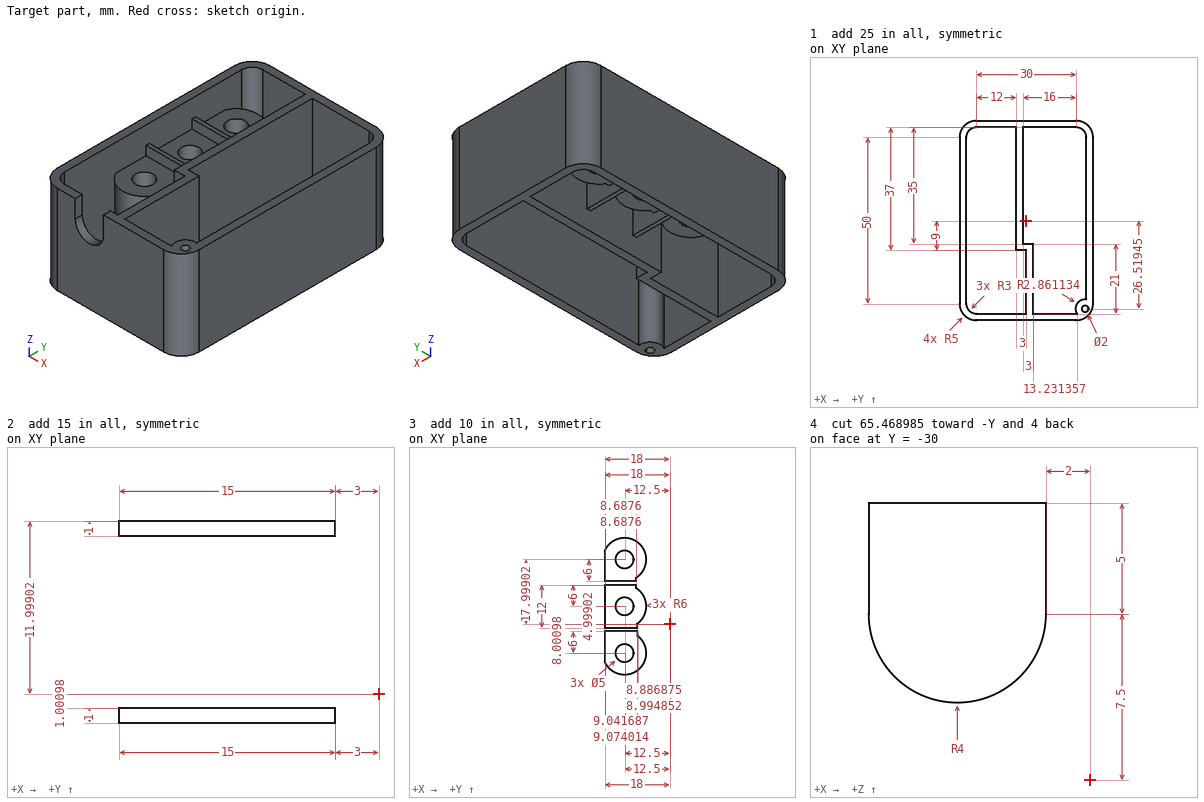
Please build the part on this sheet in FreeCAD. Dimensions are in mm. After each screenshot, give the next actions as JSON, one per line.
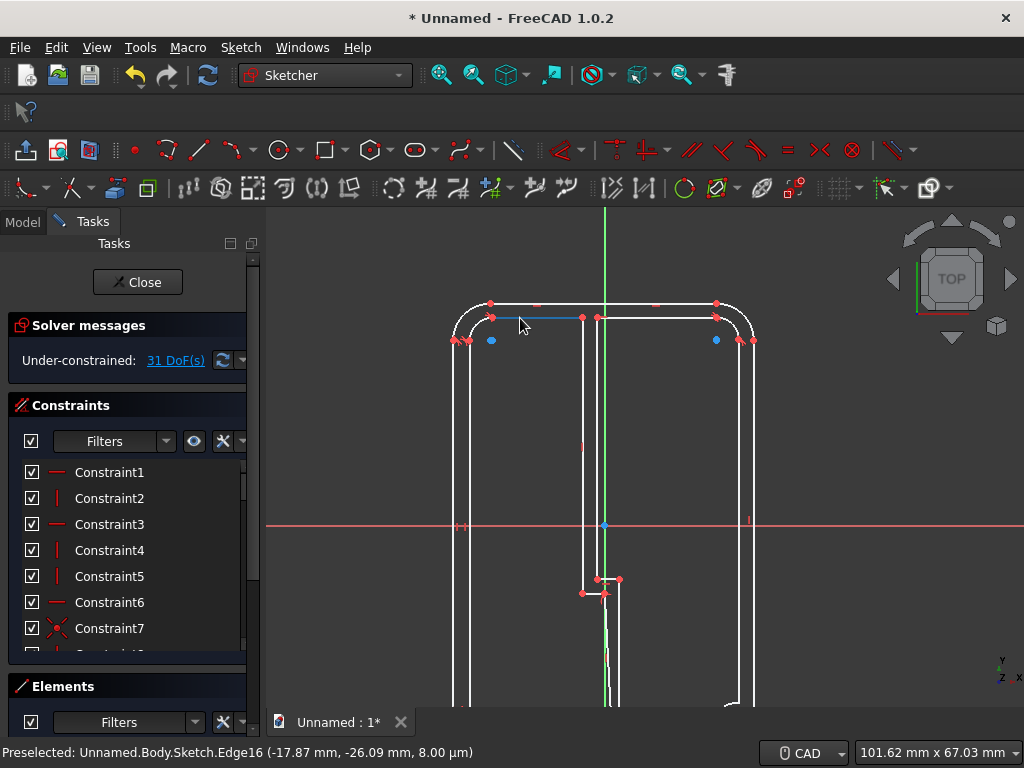
{"action": "left_click", "coordinate": [519, 318]}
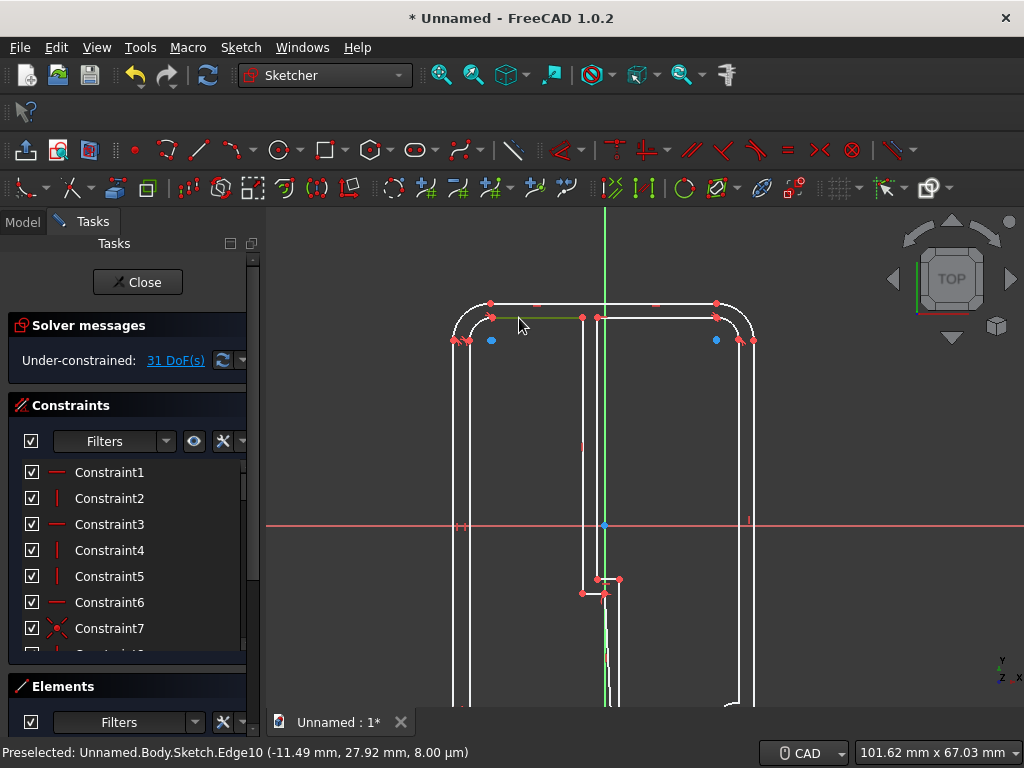
{"action": "scroll", "coordinate": [482, 320], "scroll_direction": "up", "scroll_amount": 2}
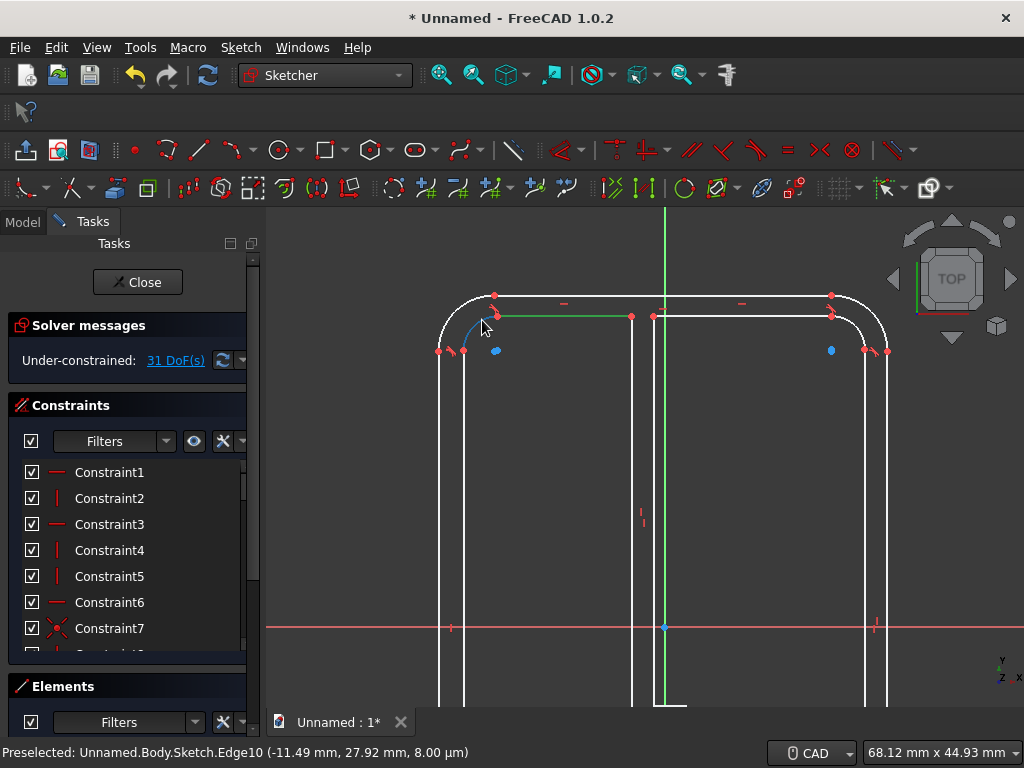
{"action": "left_click", "coordinate": [482, 320]}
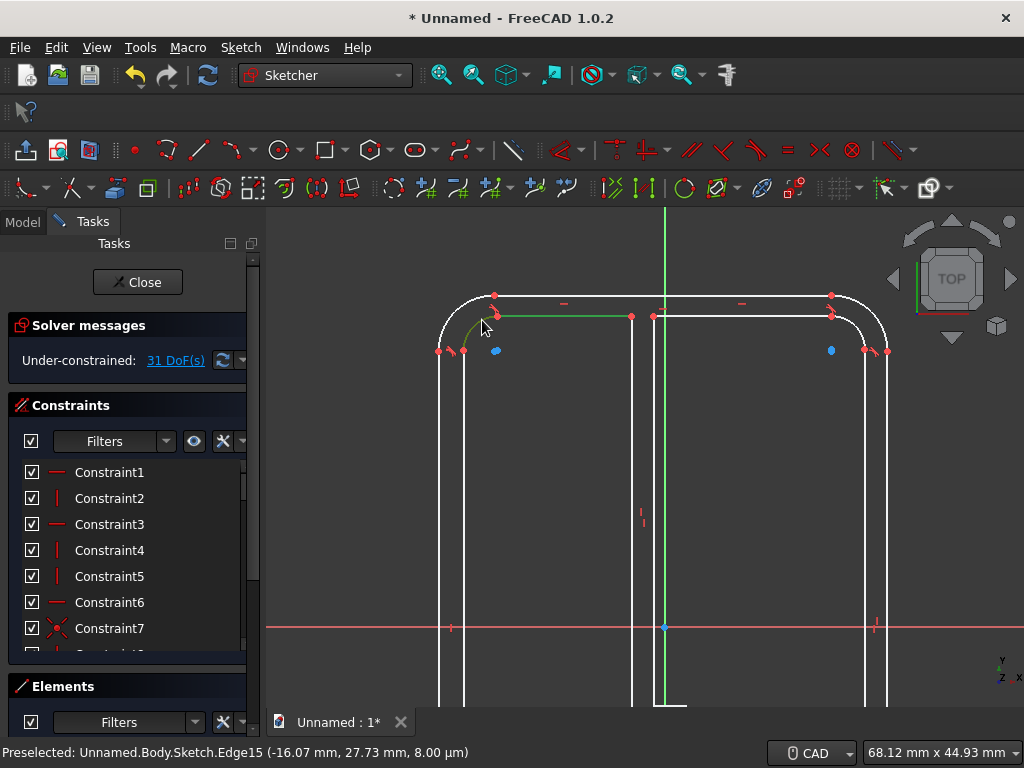
{"action": "left_click", "coordinate": [756, 150]}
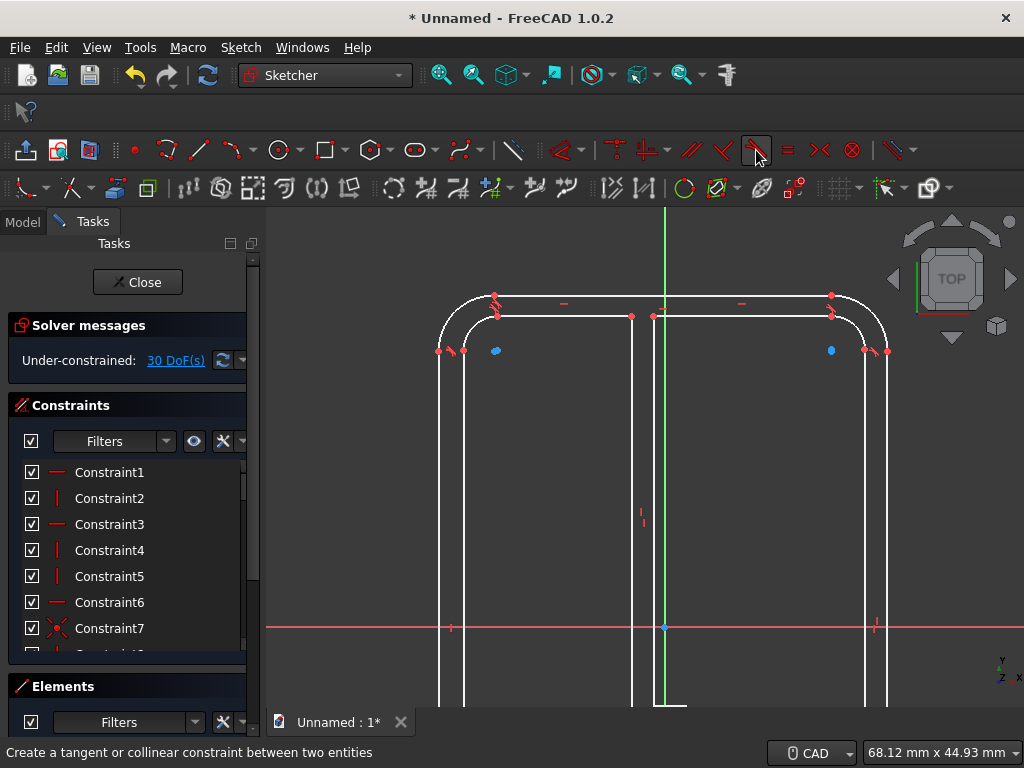
{"action": "scroll", "coordinate": [504, 318], "scroll_direction": "down", "scroll_amount": 4}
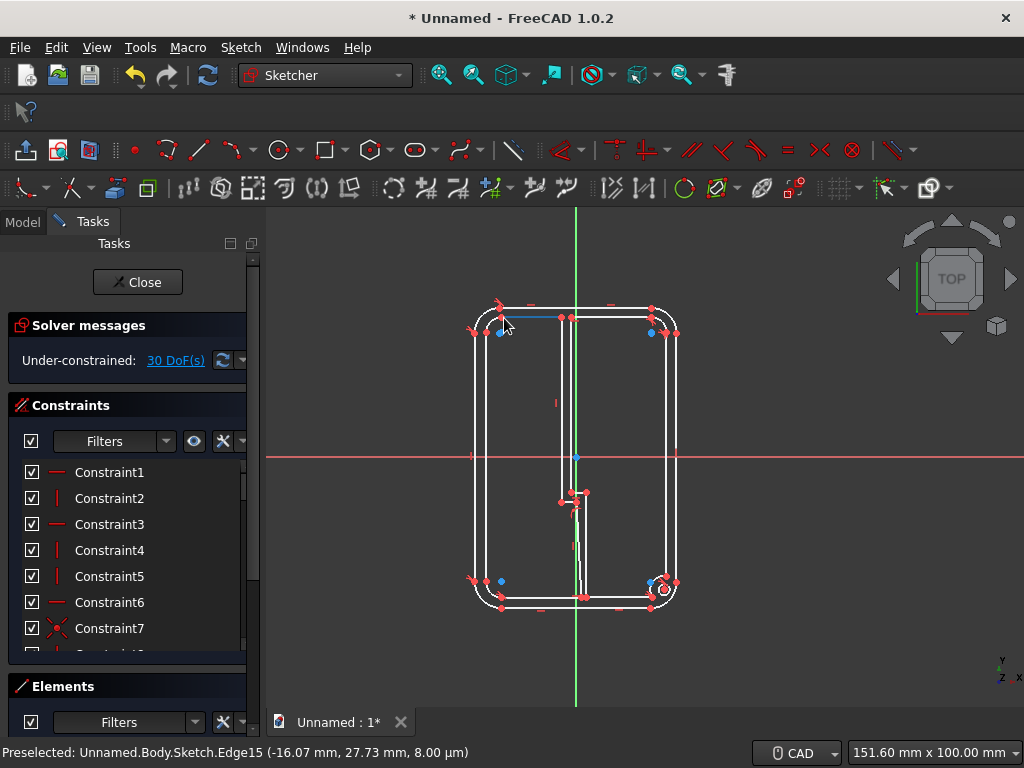
{"action": "scroll", "coordinate": [557, 598], "scroll_direction": "up", "scroll_amount": 2}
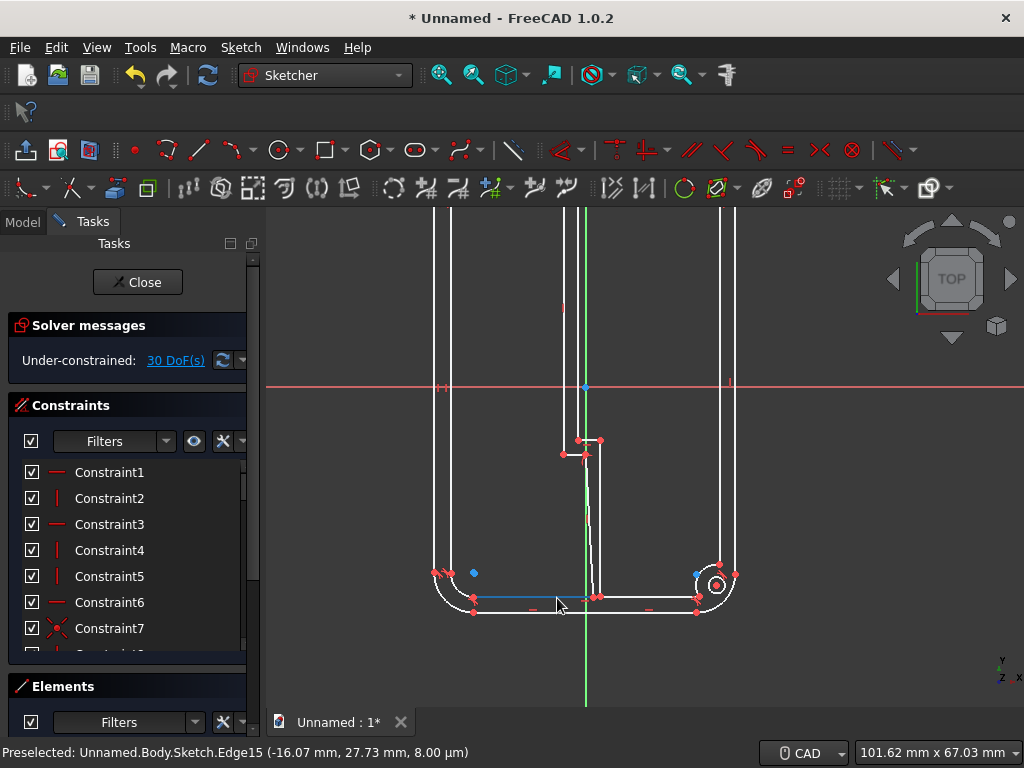
{"action": "left_click", "coordinate": [557, 597]}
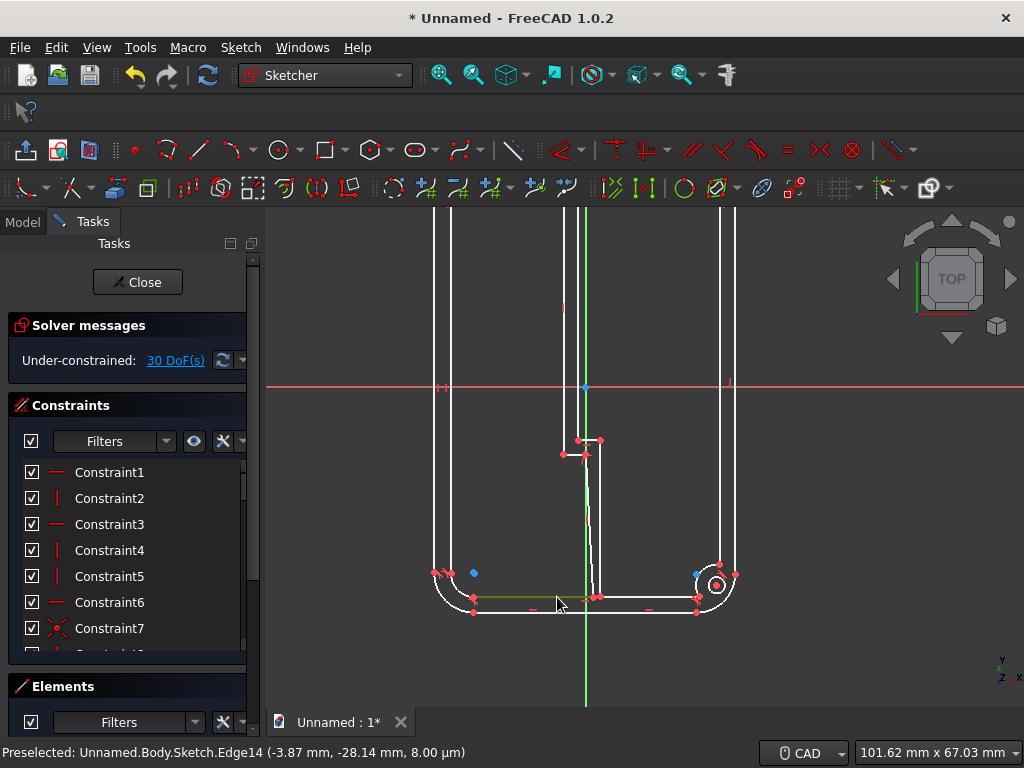
{"action": "scroll", "coordinate": [453, 584], "scroll_direction": "up", "scroll_amount": 2}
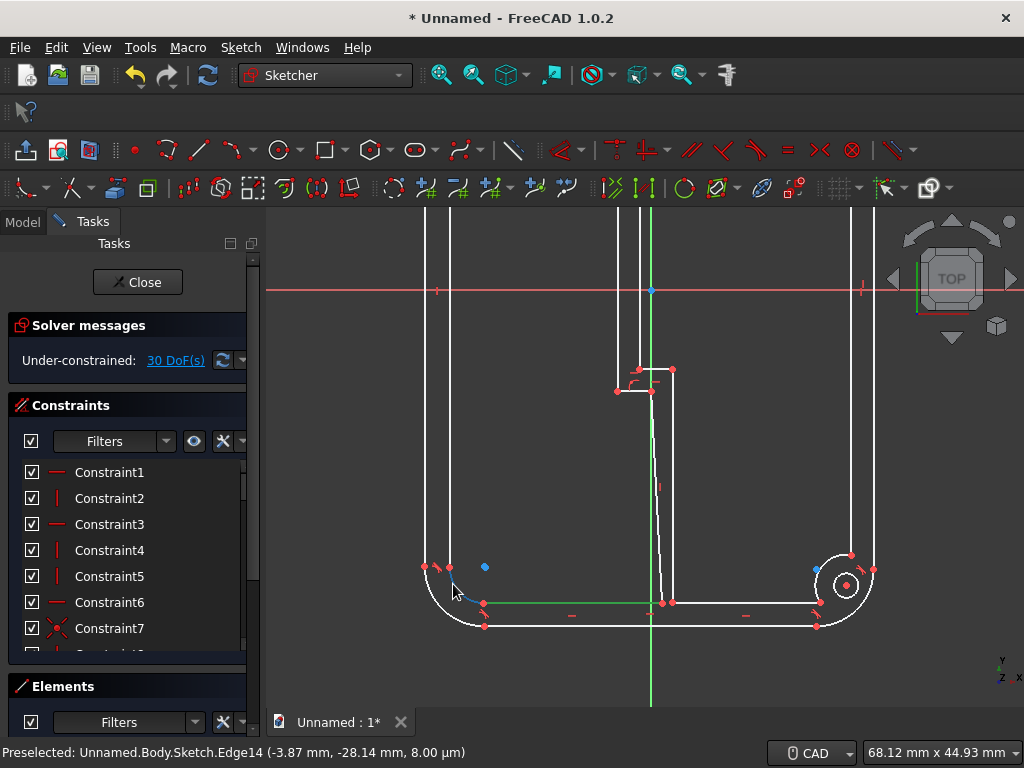
{"action": "left_click", "coordinate": [454, 584]}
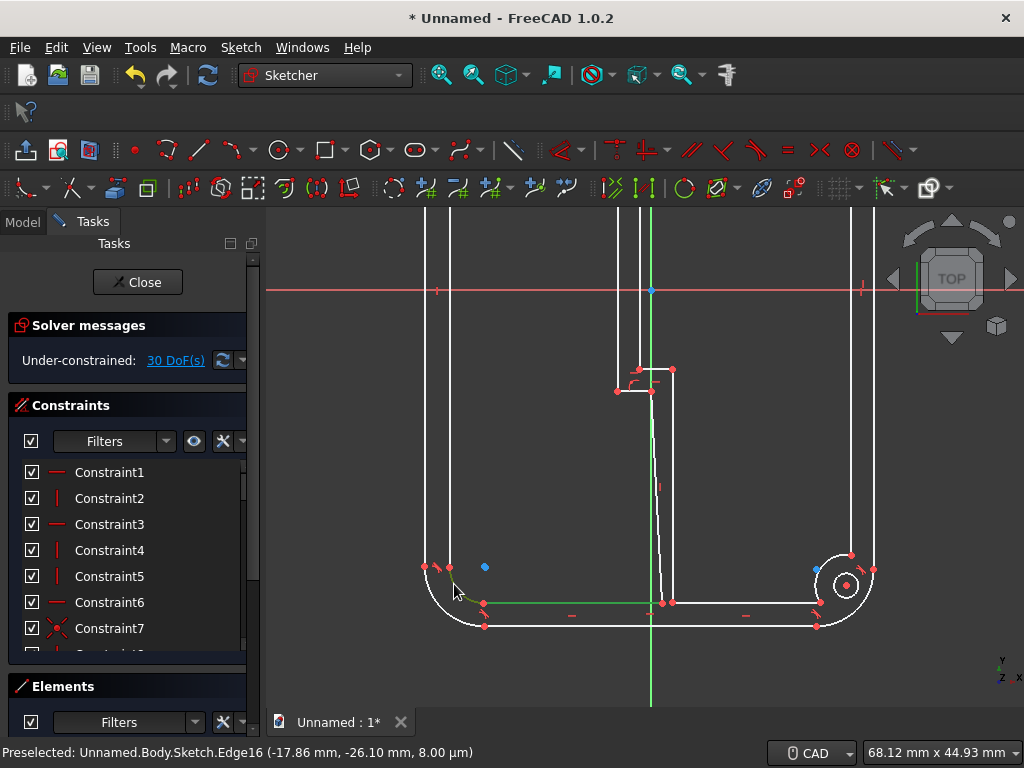
{"action": "left_click", "coordinate": [756, 150]}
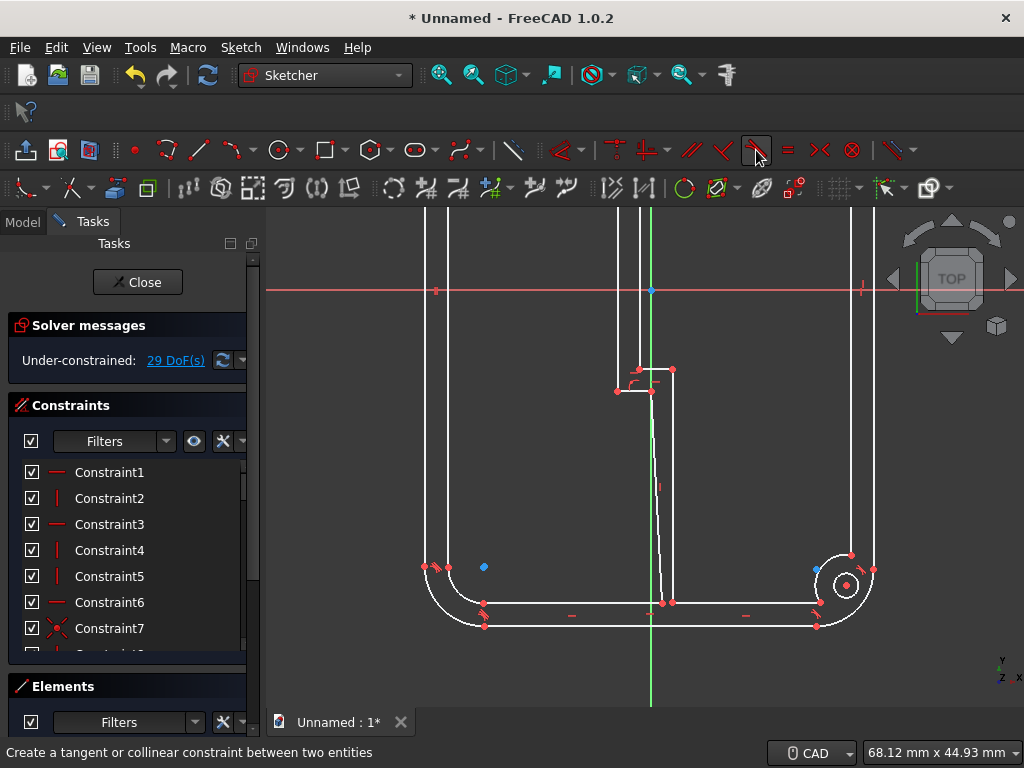
{"action": "left_click", "coordinate": [851, 392]}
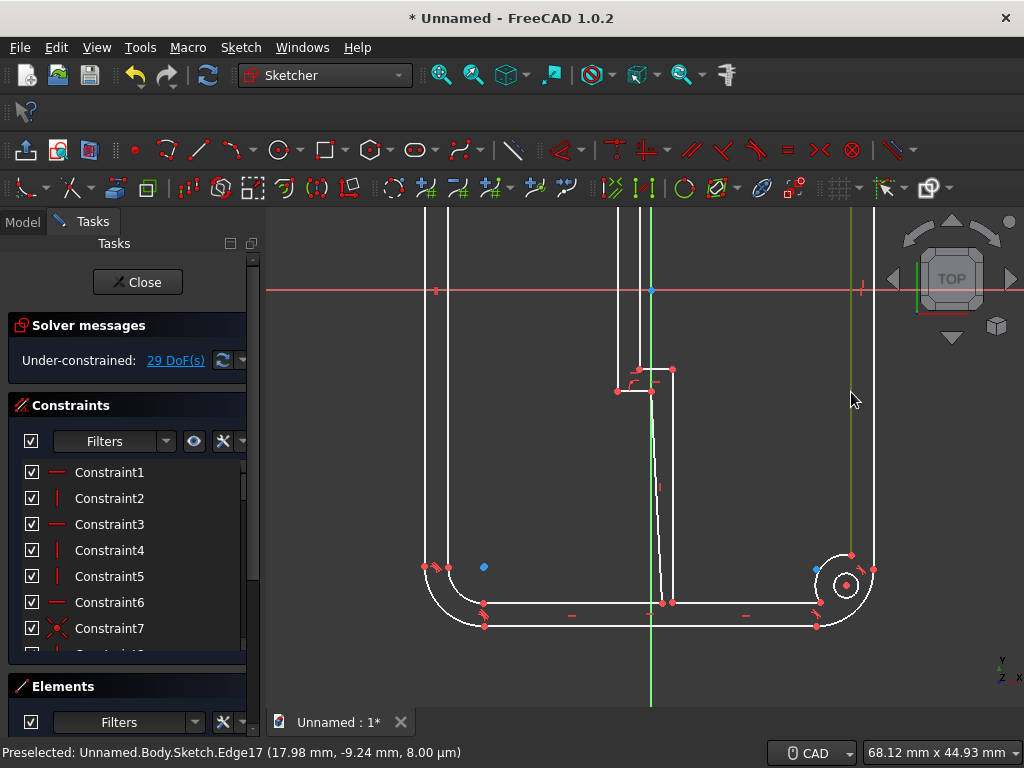
{"action": "scroll", "coordinate": [516, 593], "scroll_direction": "down", "scroll_amount": 4}